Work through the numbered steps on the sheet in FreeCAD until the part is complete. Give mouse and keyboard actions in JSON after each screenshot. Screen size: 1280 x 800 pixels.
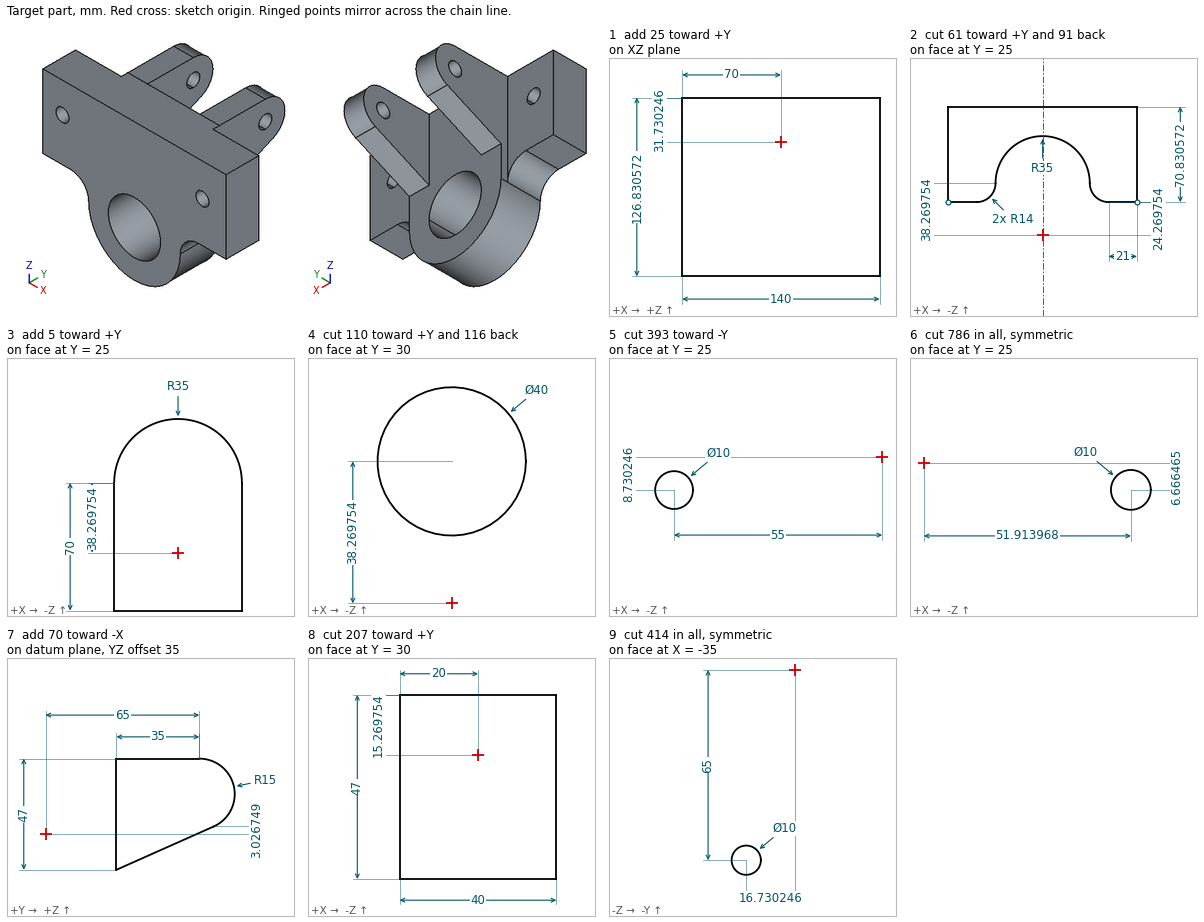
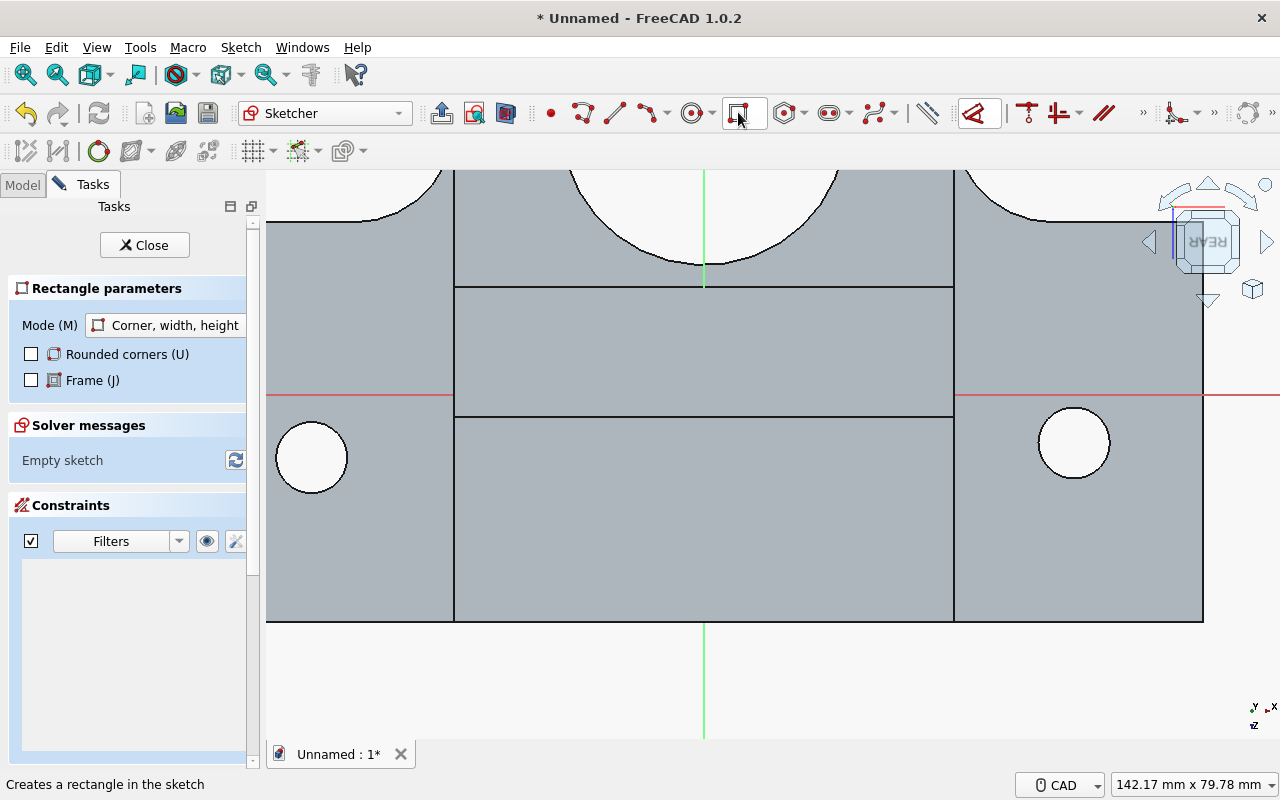
{"action": "left_click", "coordinate": [561, 287]}
{"action": "left_click", "coordinate": [847, 622]}
{"action": "key", "text": "Escape"}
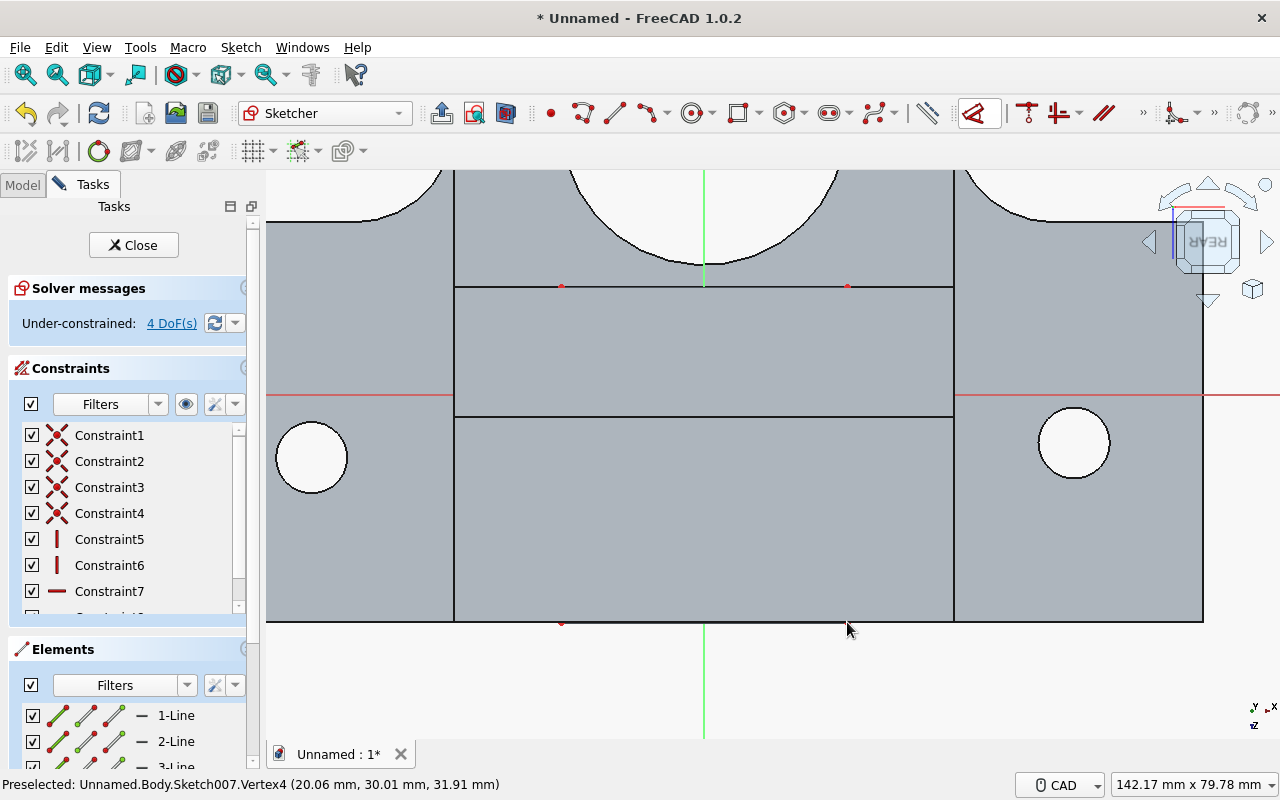
{"action": "left_click", "coordinate": [561, 522]}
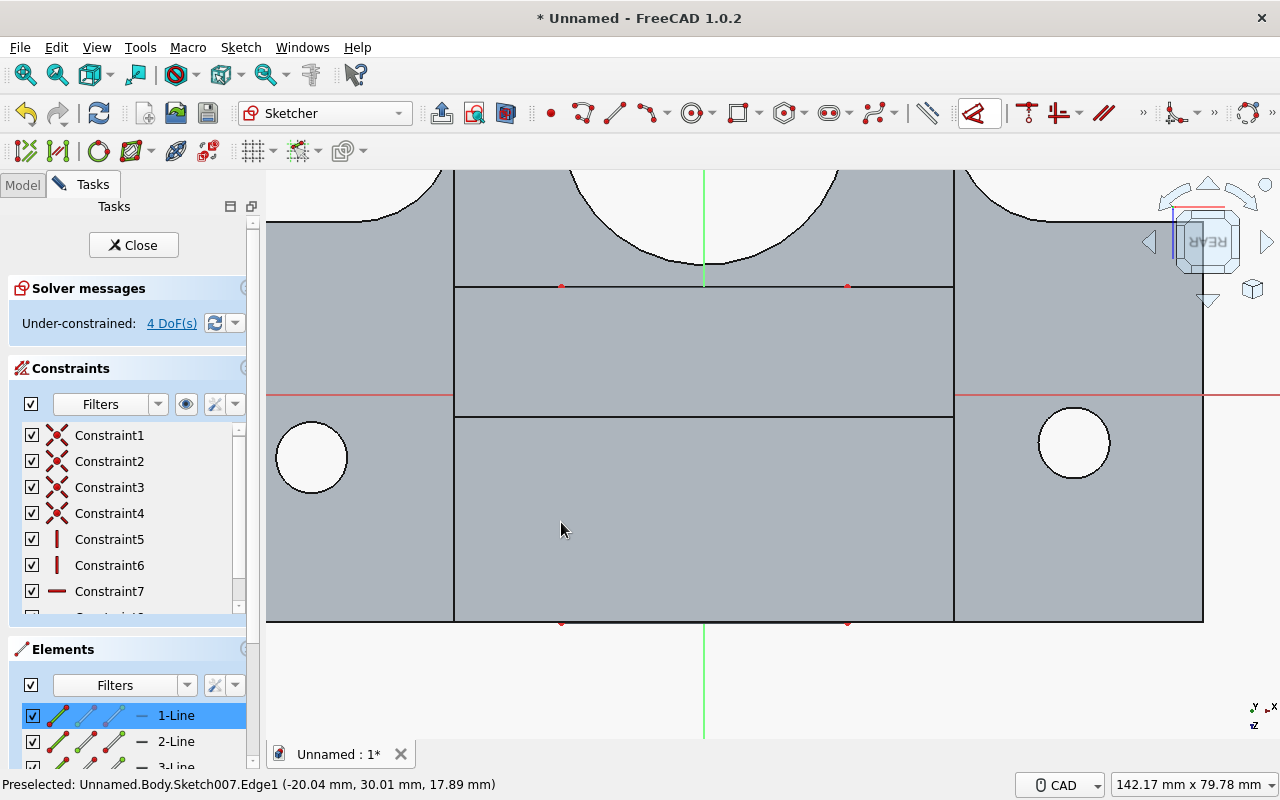
{"action": "left_click", "coordinate": [996, 114]}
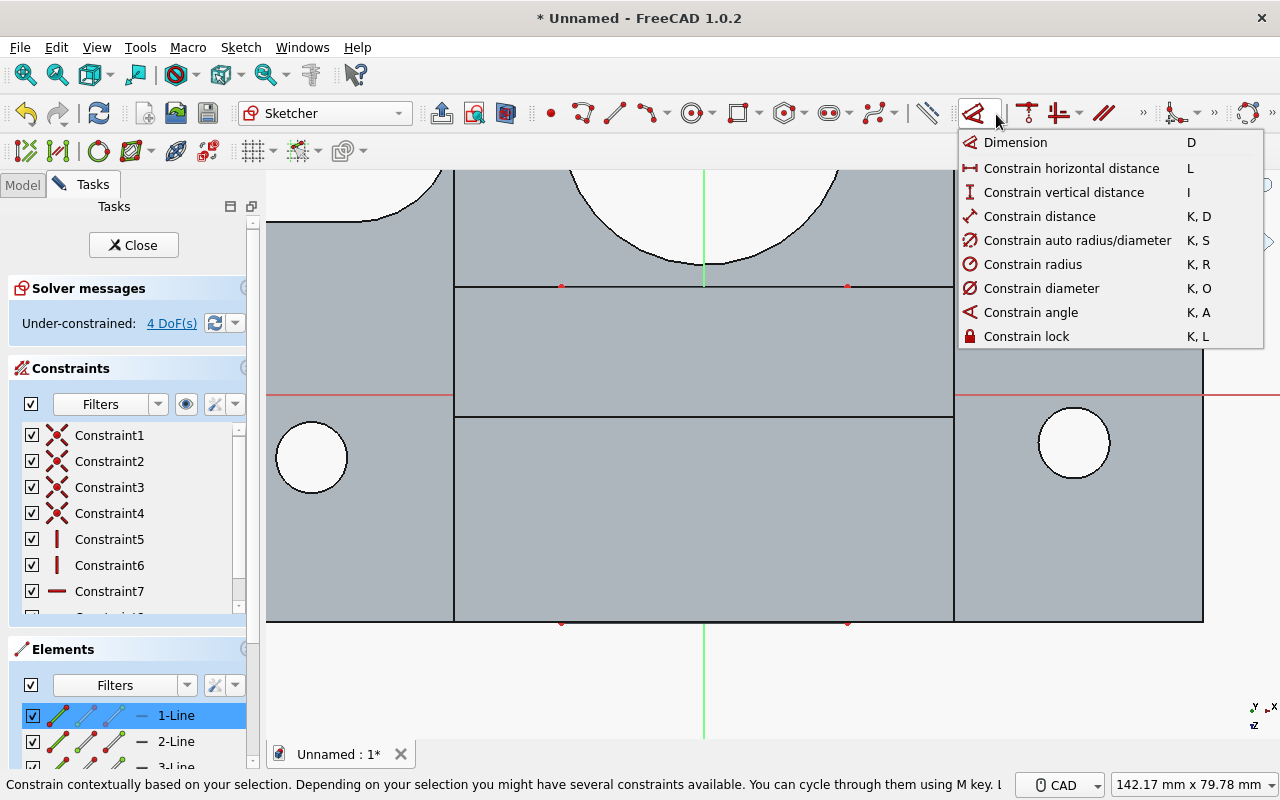
{"action": "left_click", "coordinate": [1111, 192]}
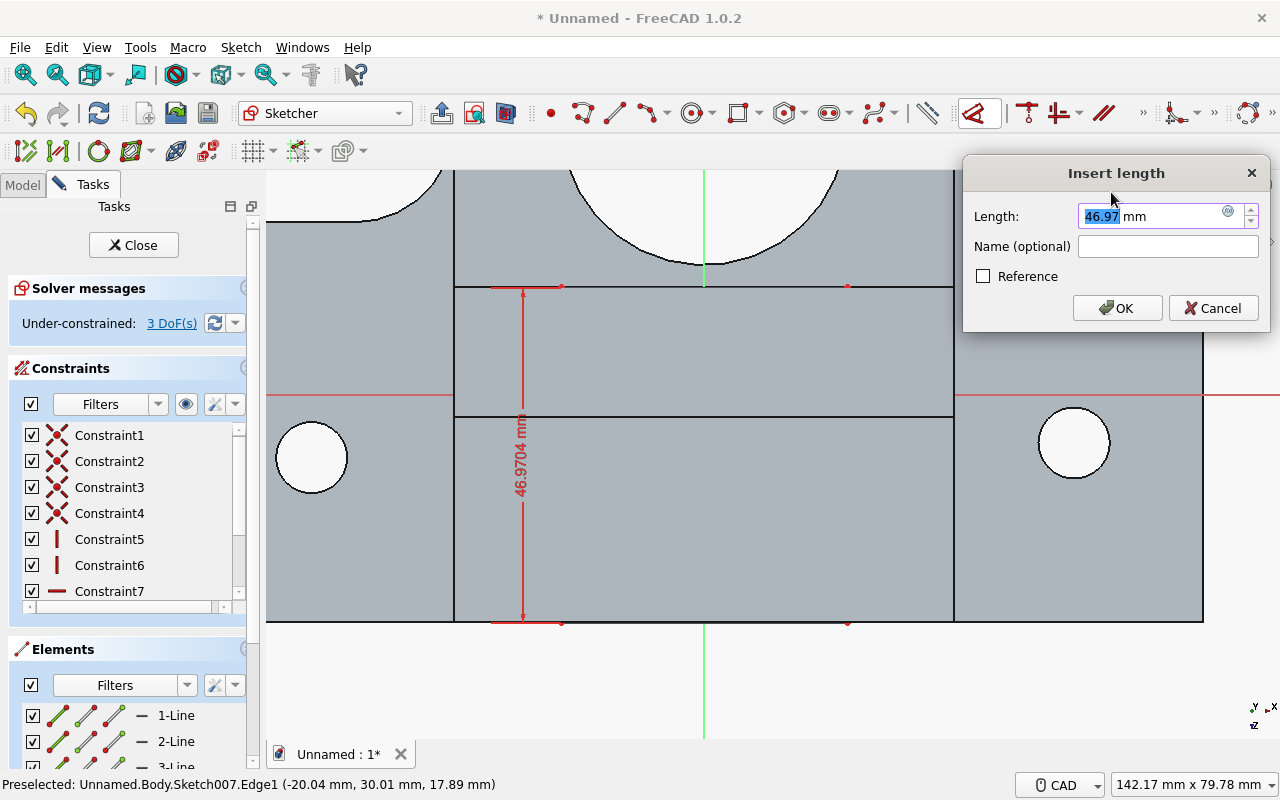
{"action": "type", "text": "47"}
{"action": "key", "text": "Return"}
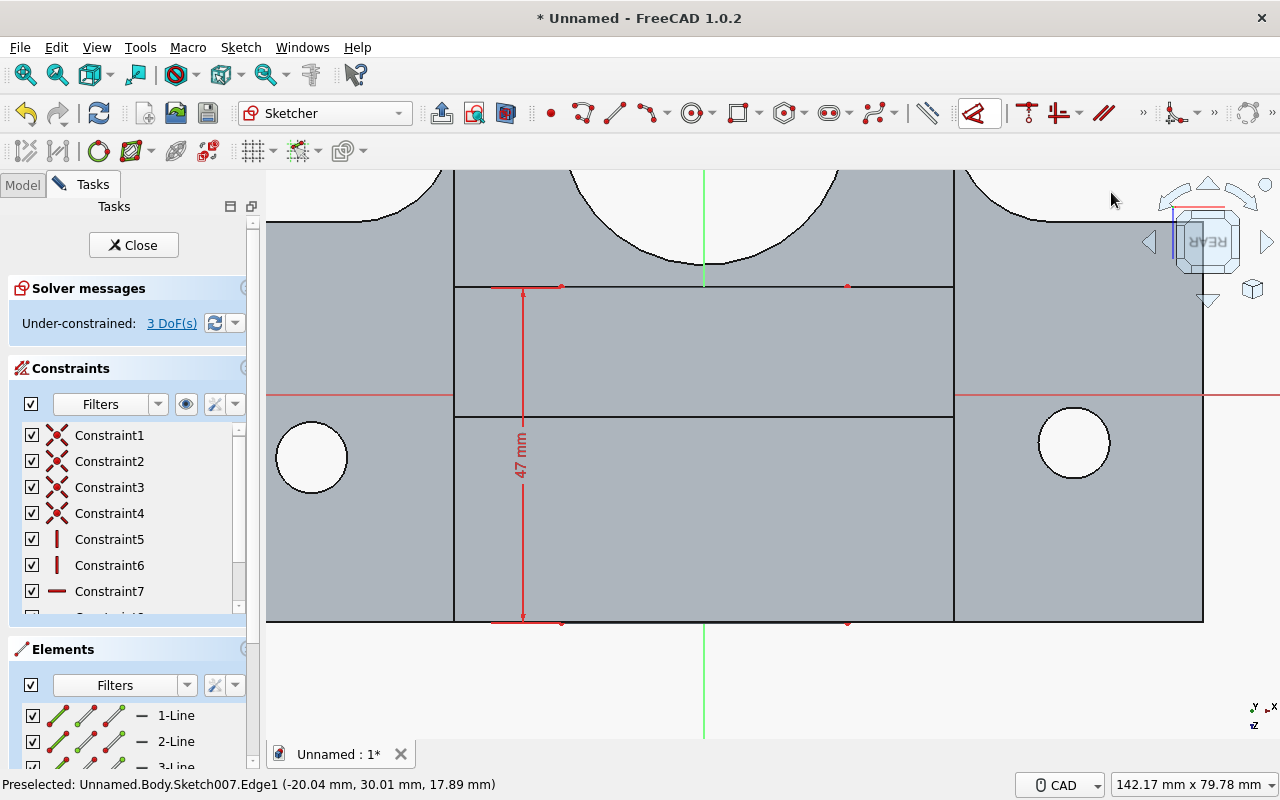
{"action": "left_click", "coordinate": [647, 623]}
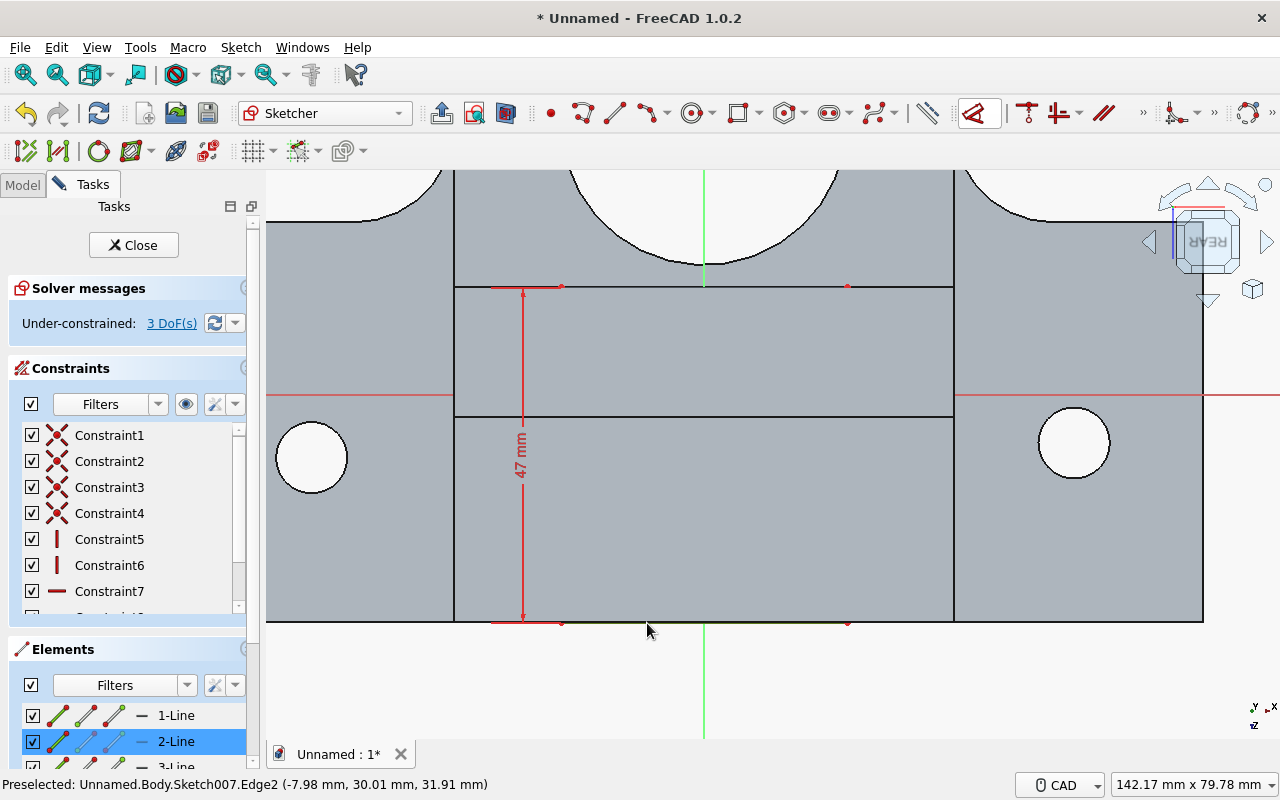
{"action": "key", "text": "l"}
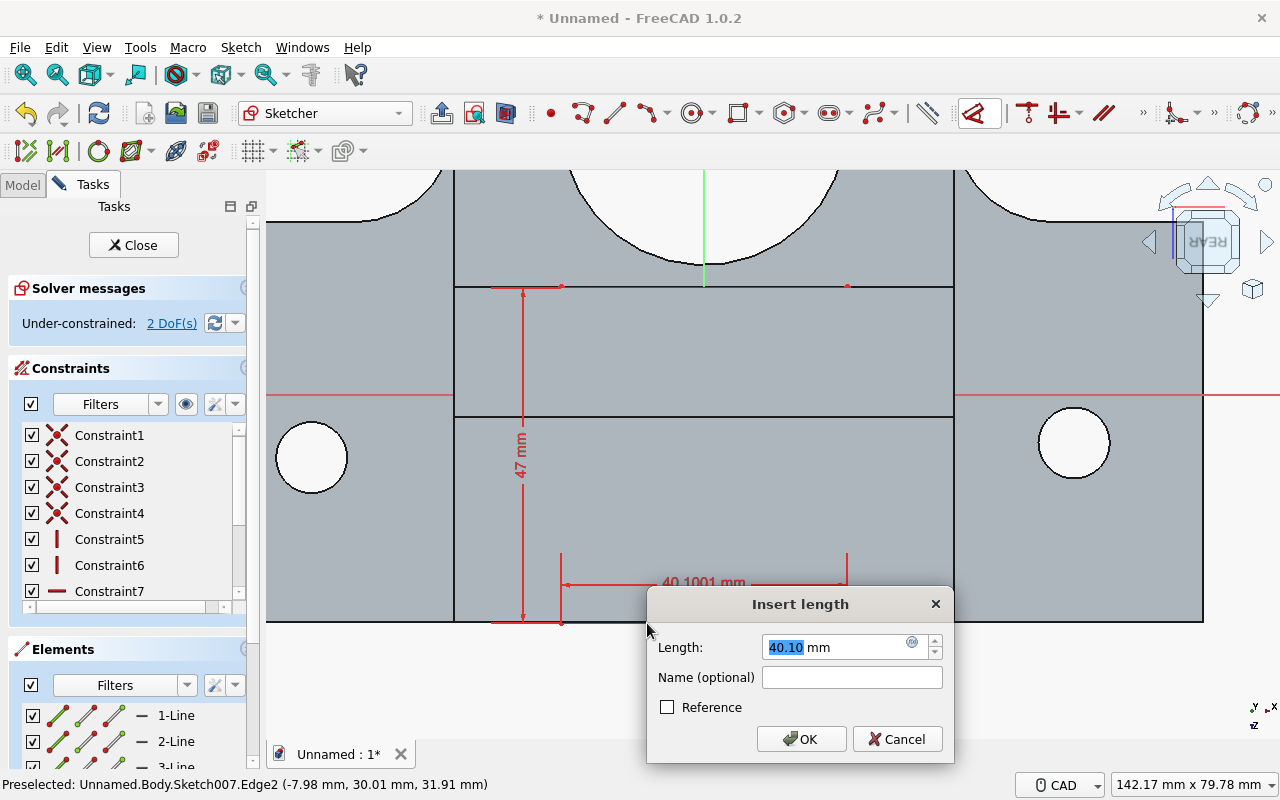
{"action": "type", "text": "40"}
{"action": "key", "text": "Return"}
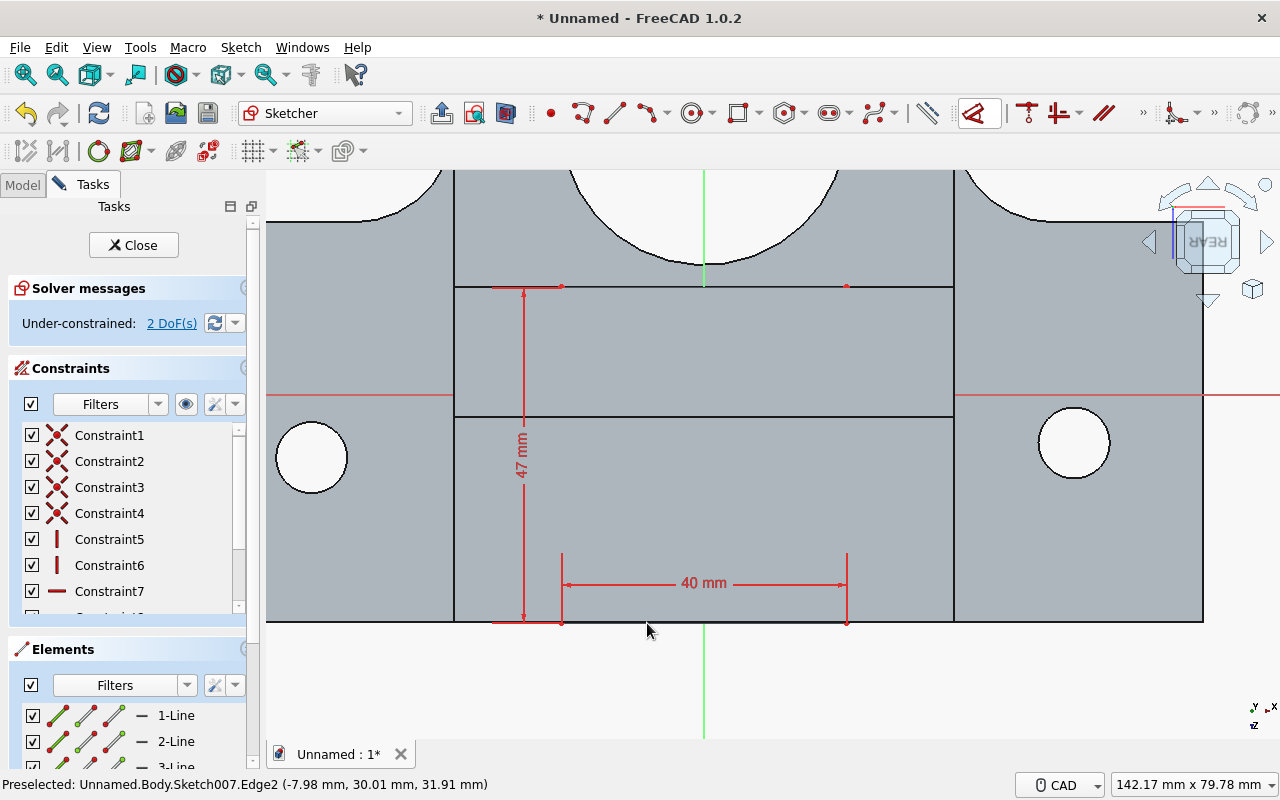
{"action": "left_click", "coordinate": [562, 288]}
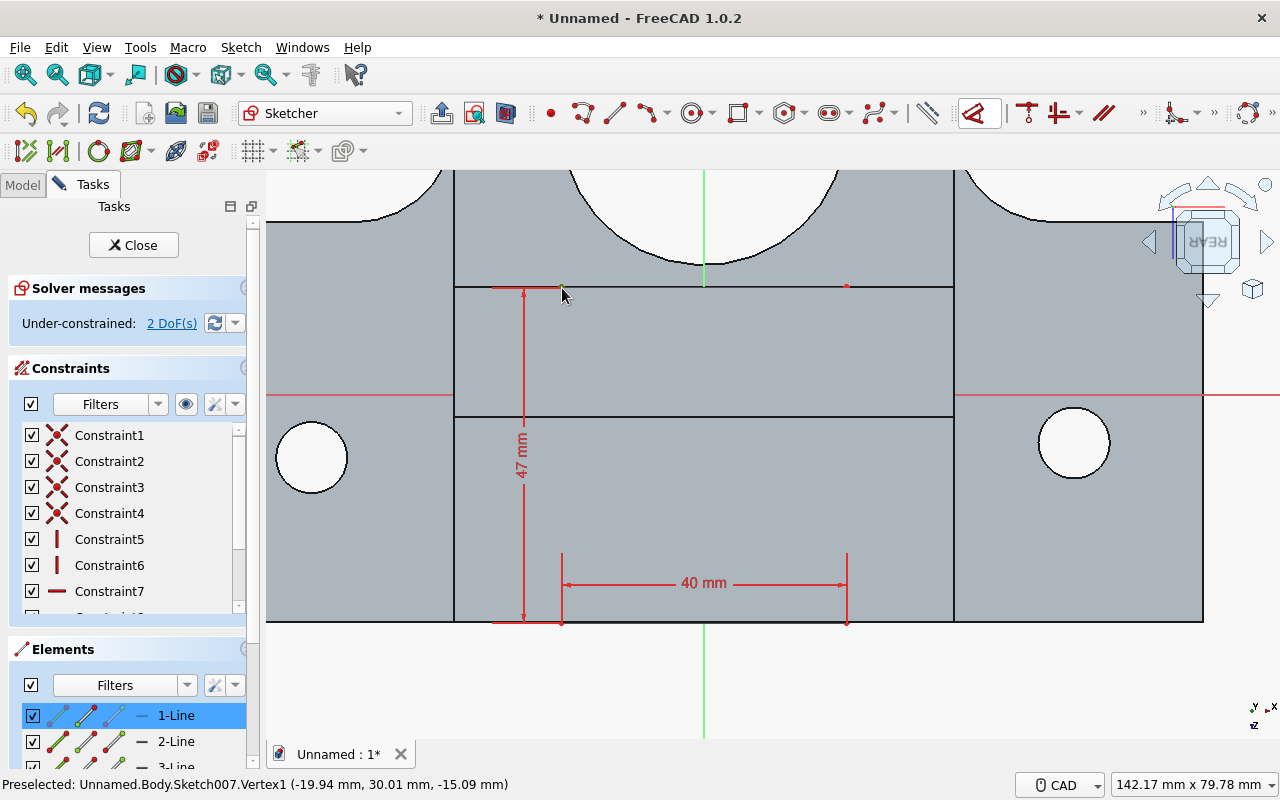
{"action": "key", "text": "l"}